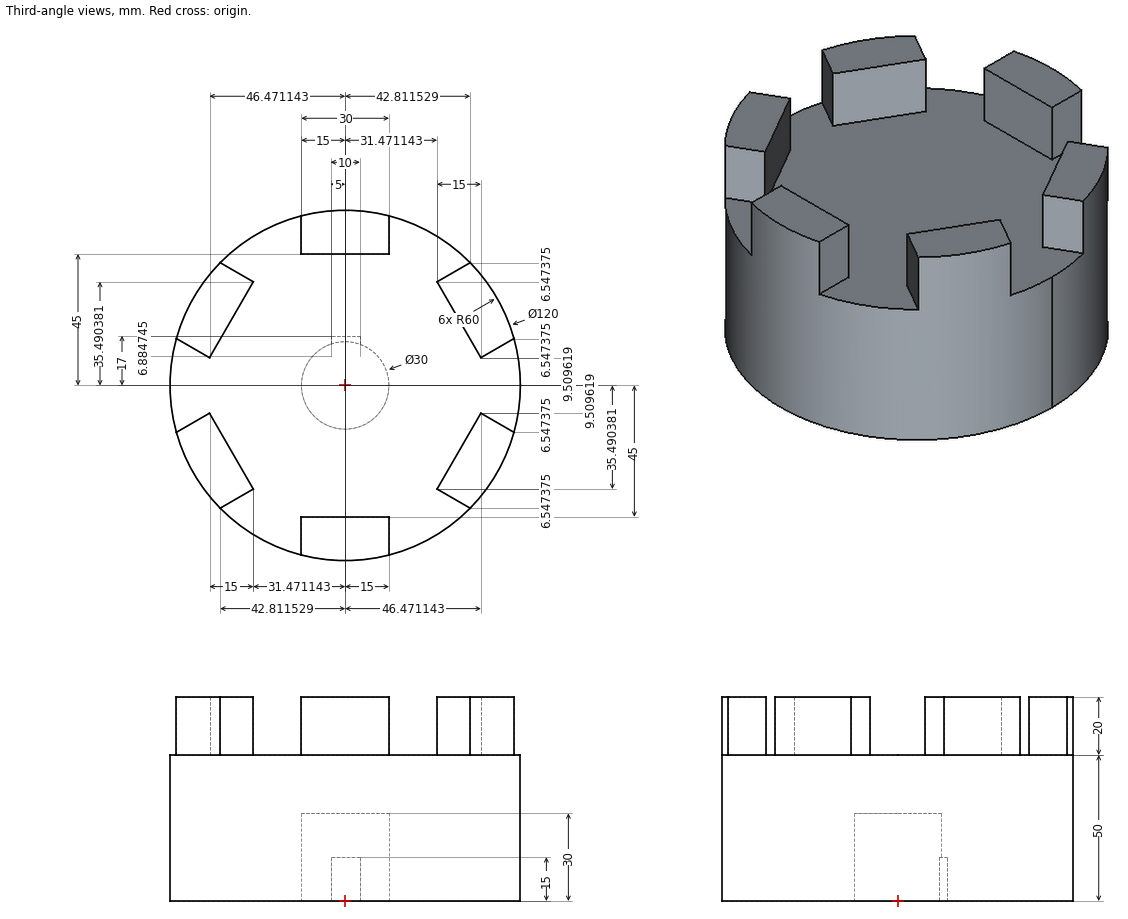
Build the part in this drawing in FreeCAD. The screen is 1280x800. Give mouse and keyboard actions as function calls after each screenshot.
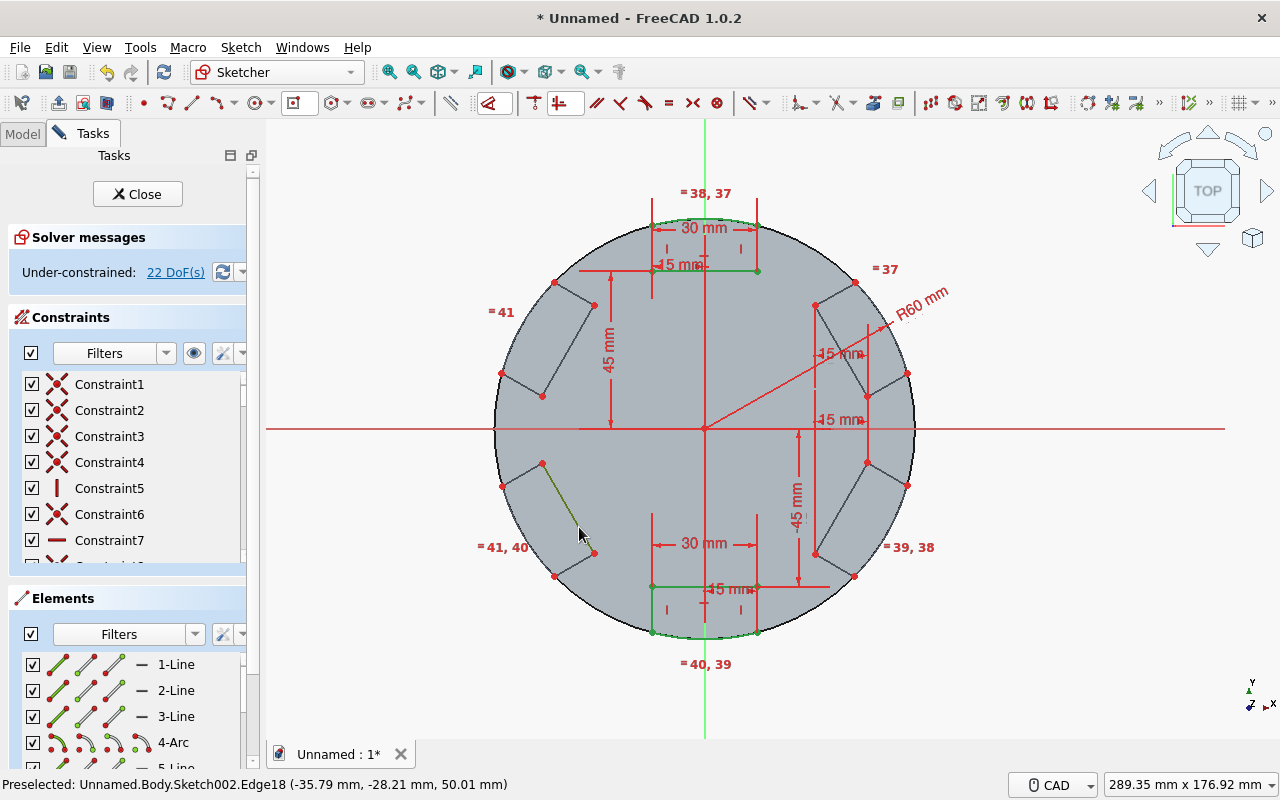
click(506, 104)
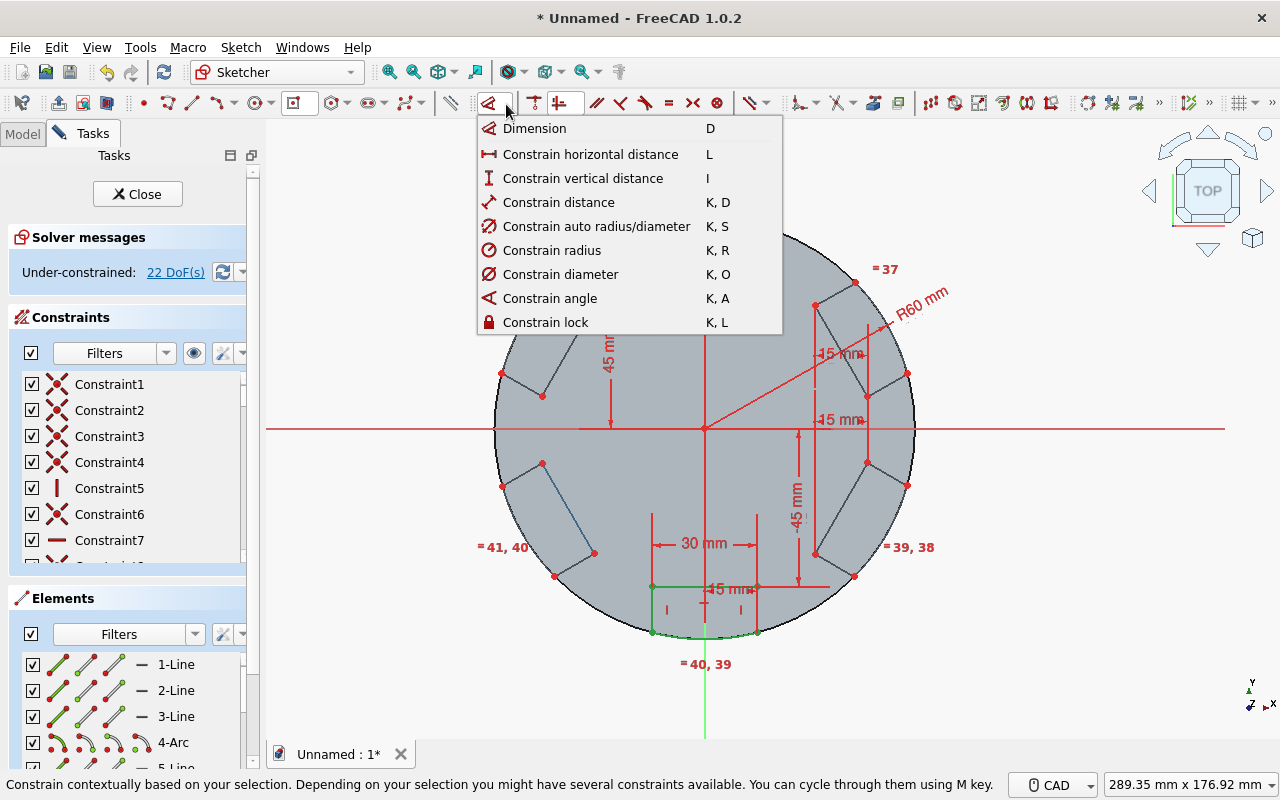
click(630, 154)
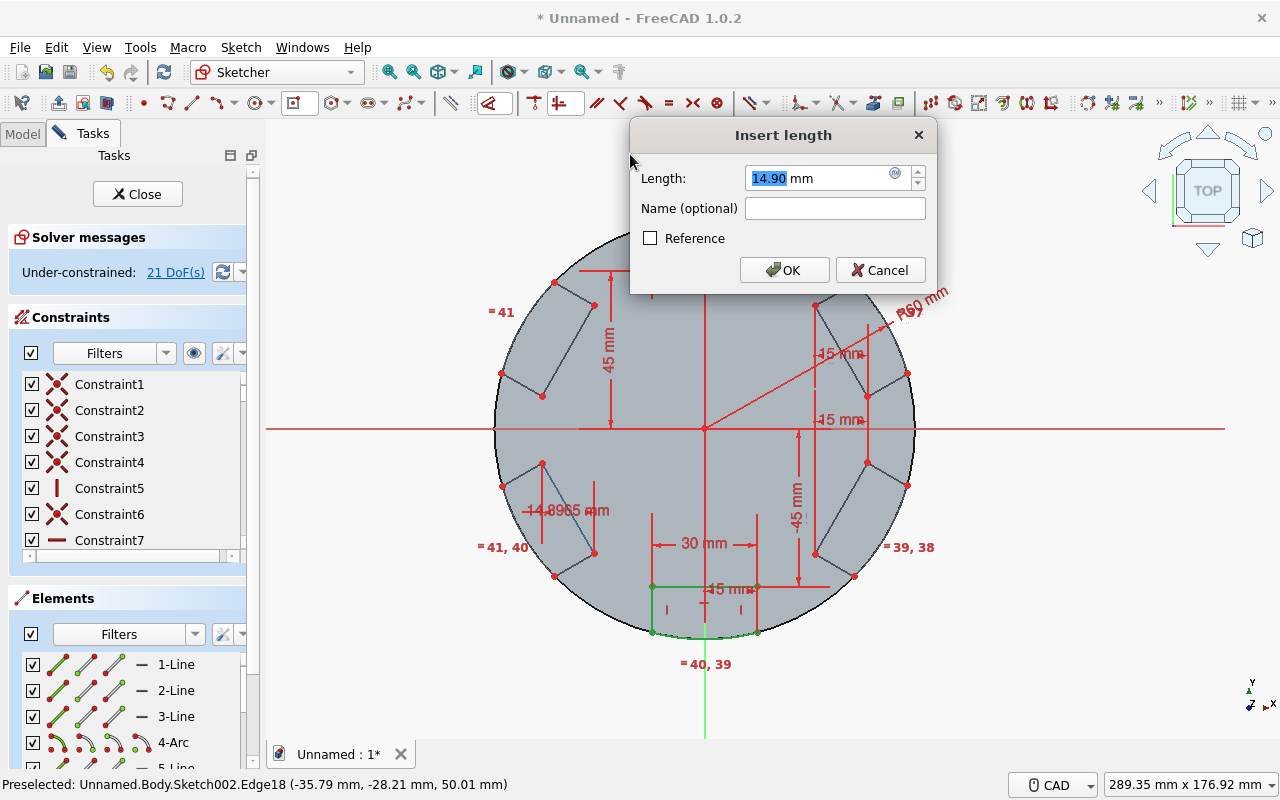
text(15)
key(Return)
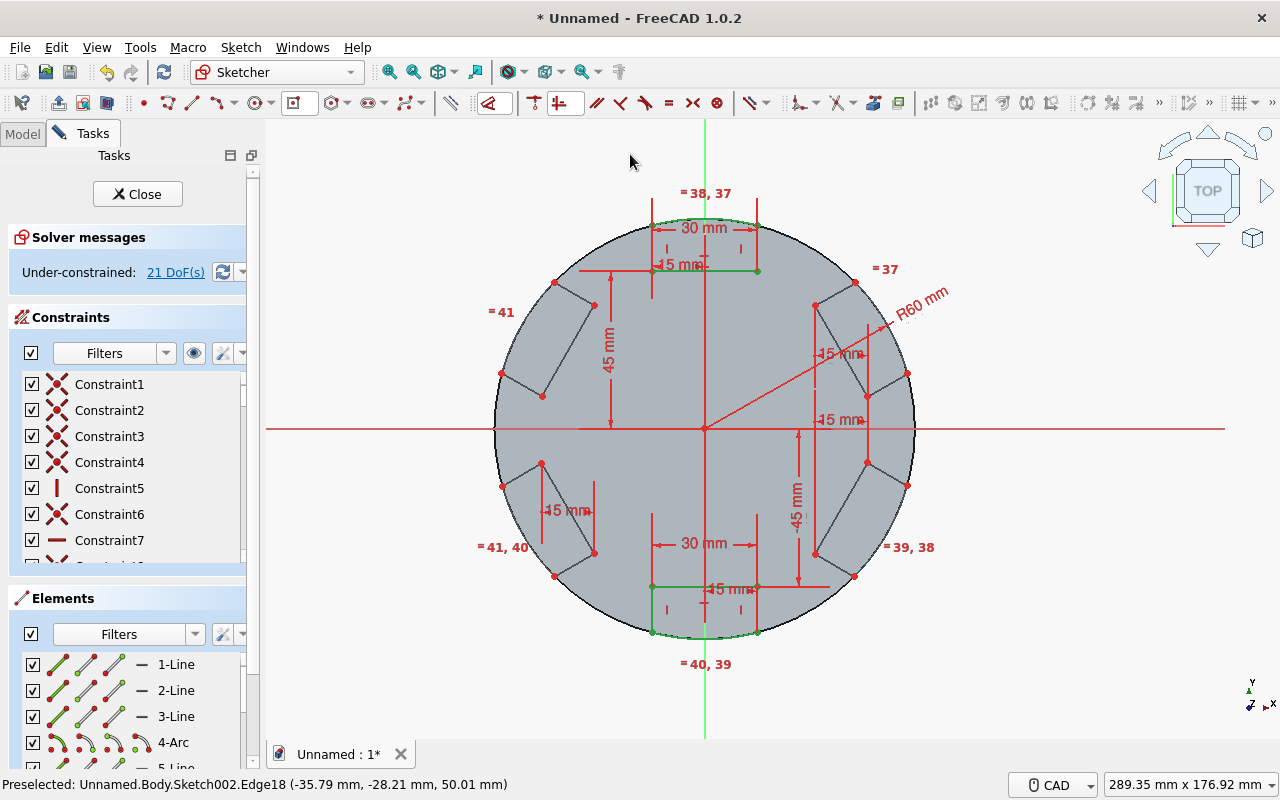
click(558, 369)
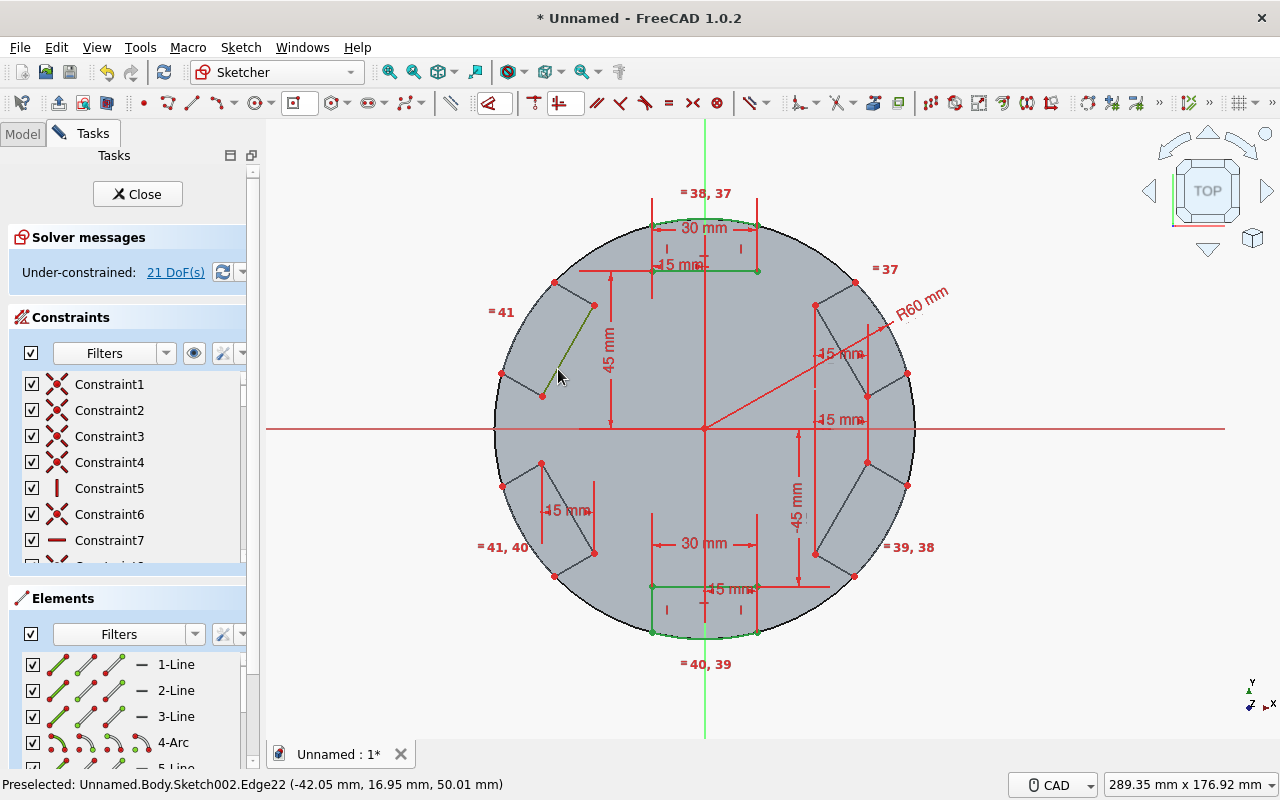
key(l)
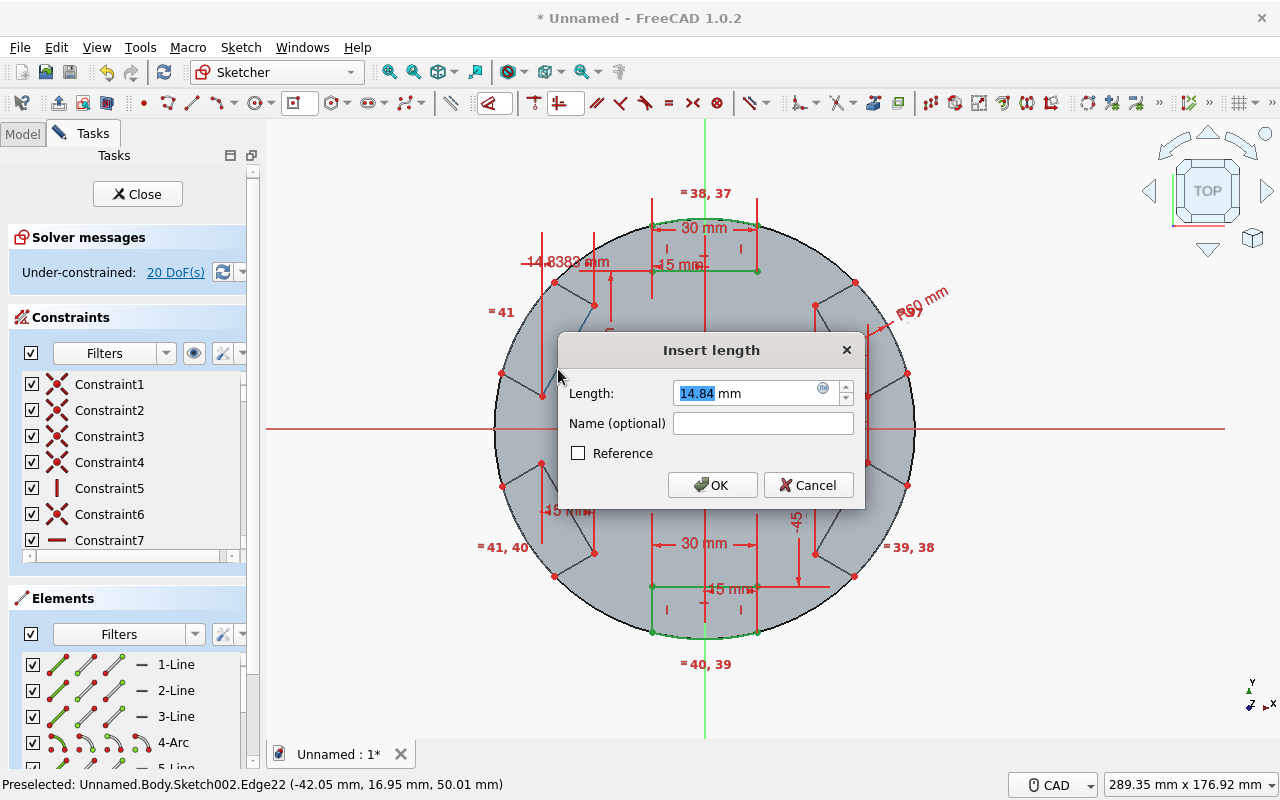
text(15)
key(Return)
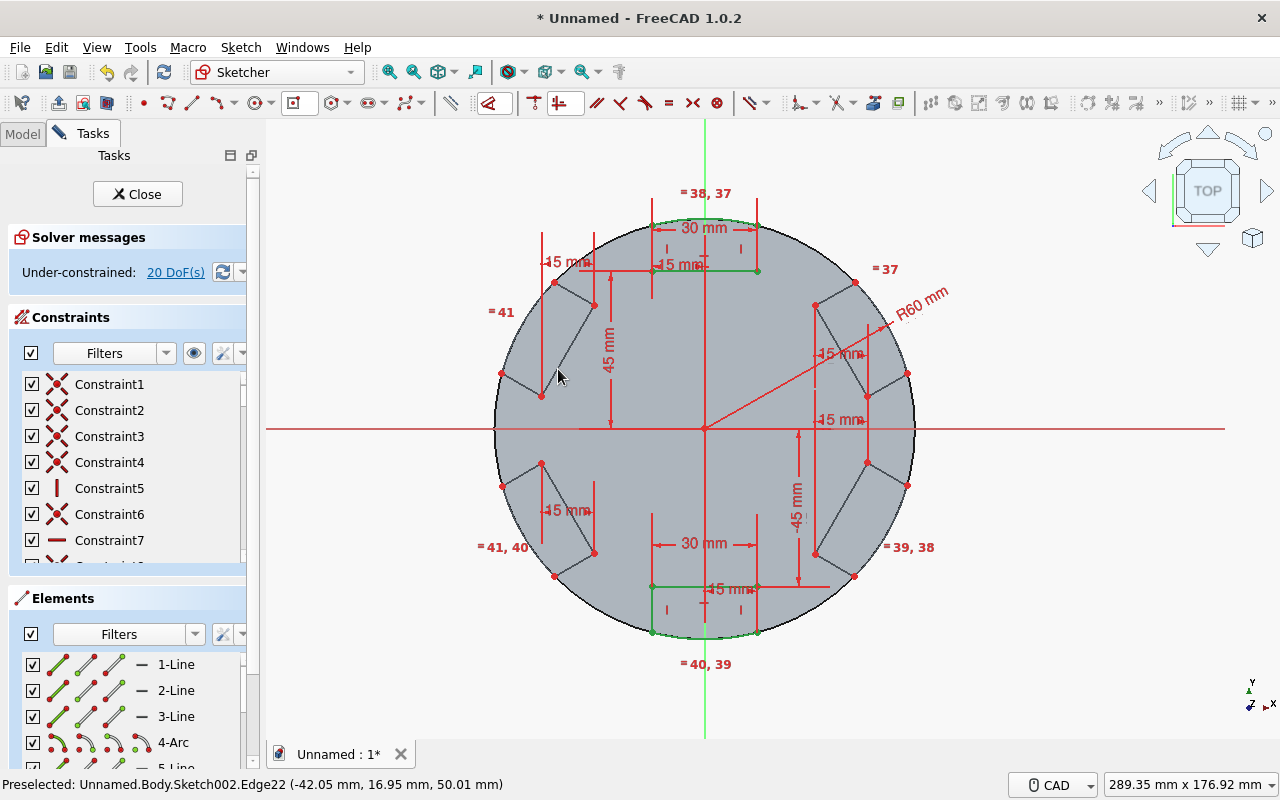
click(868, 397)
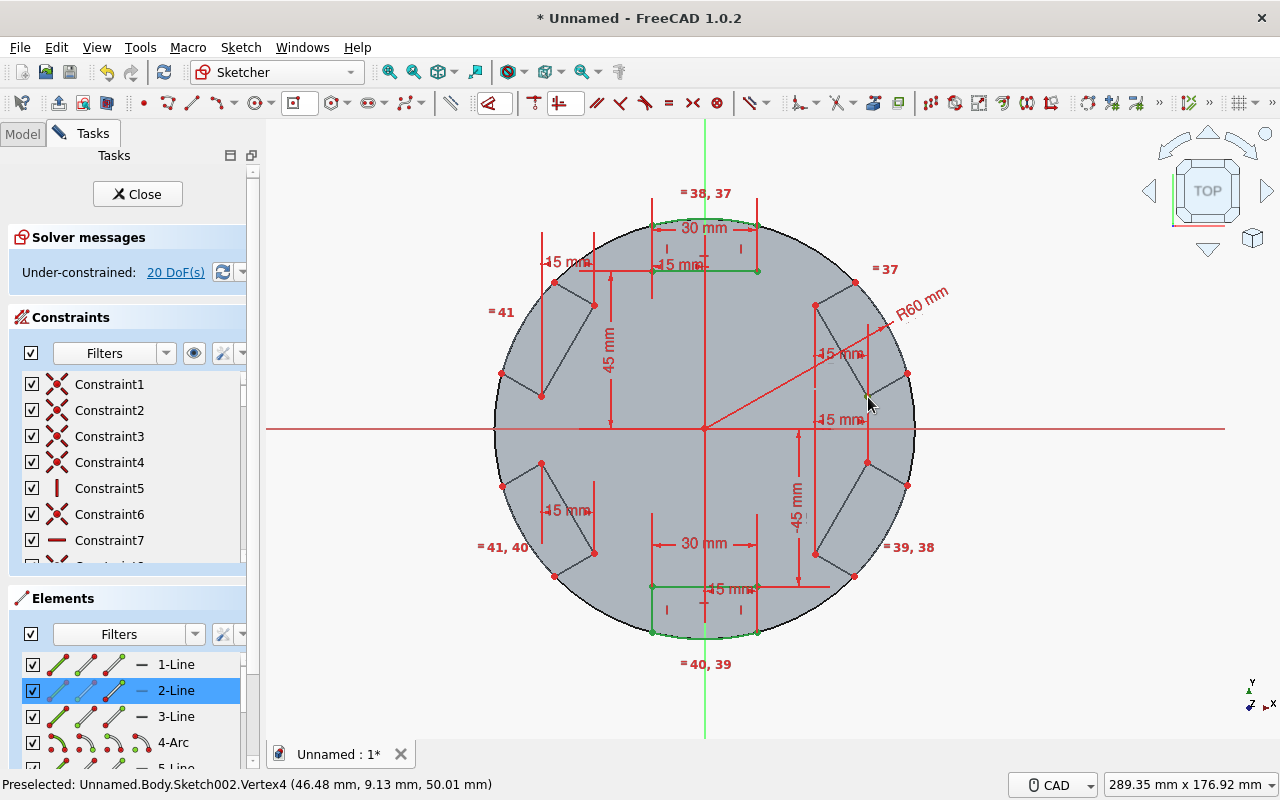
click(506, 104)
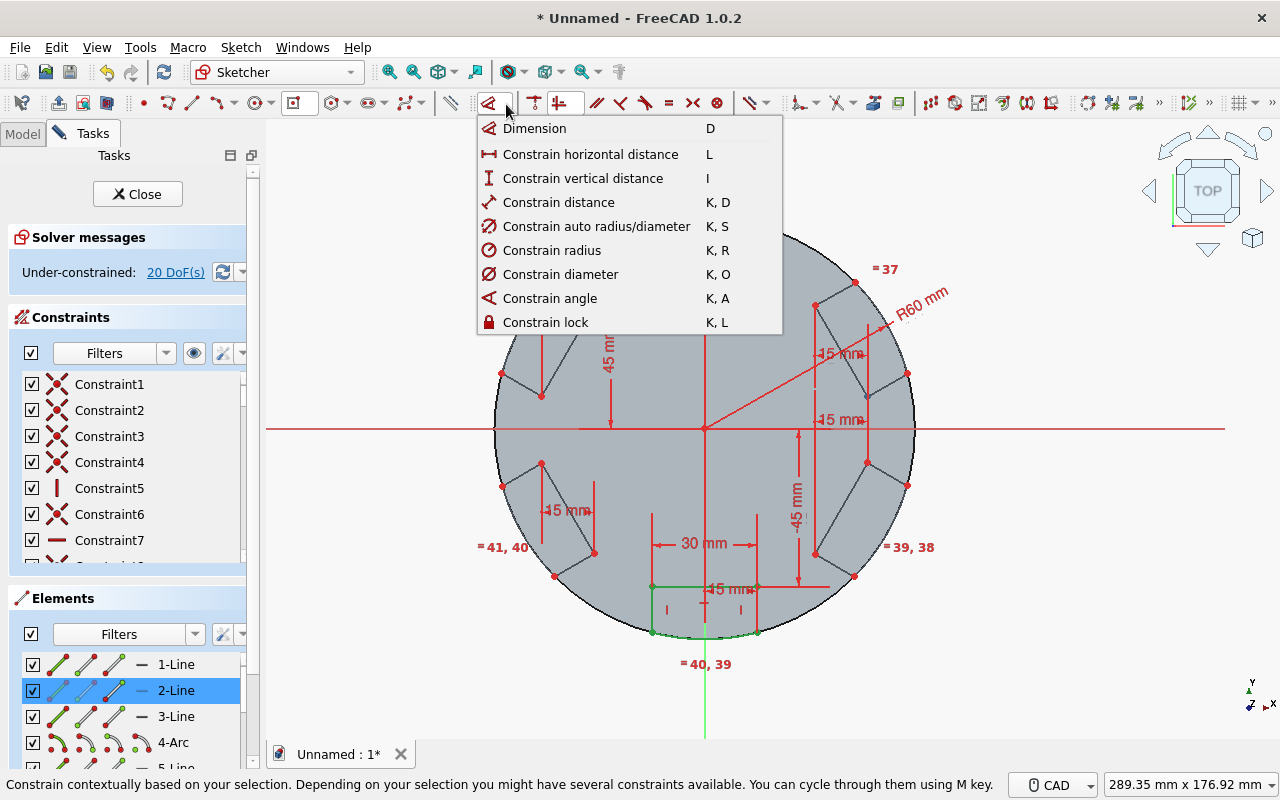
click(630, 178)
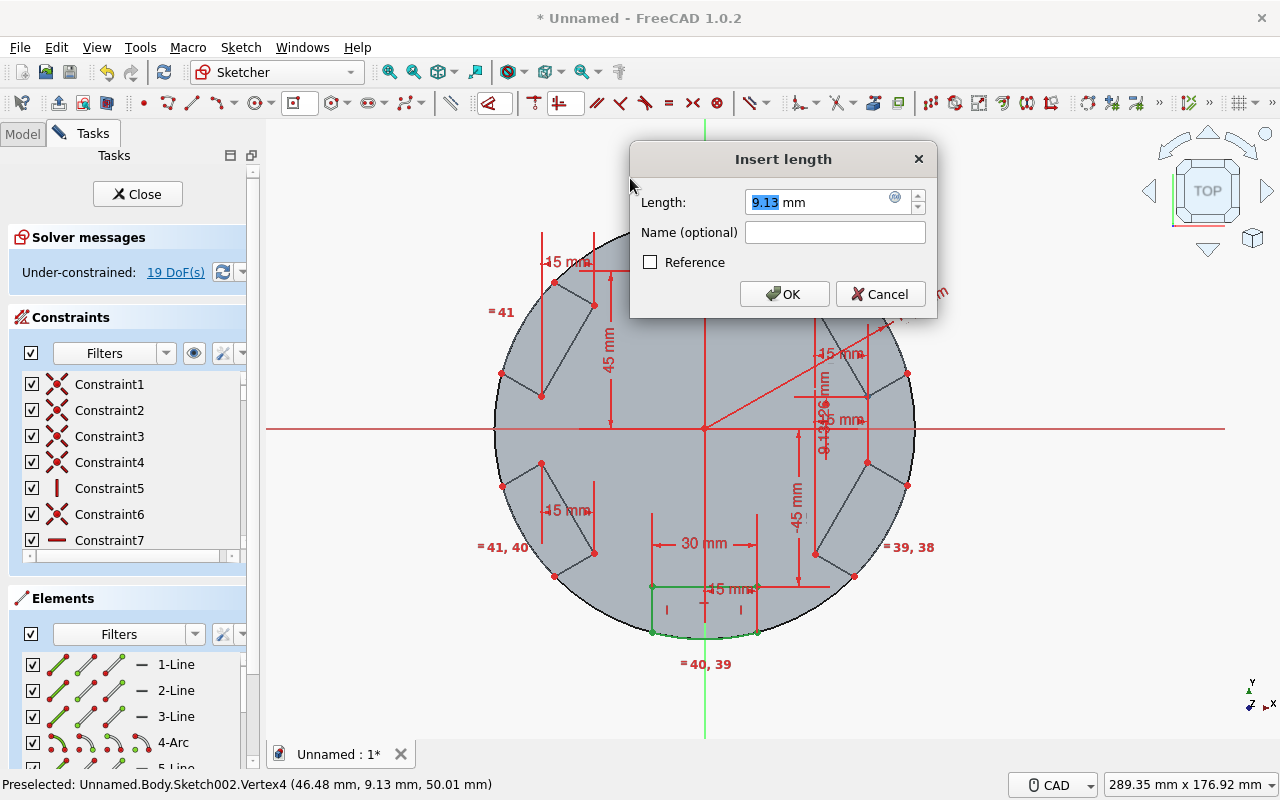
text(9.509619)
key(Return)